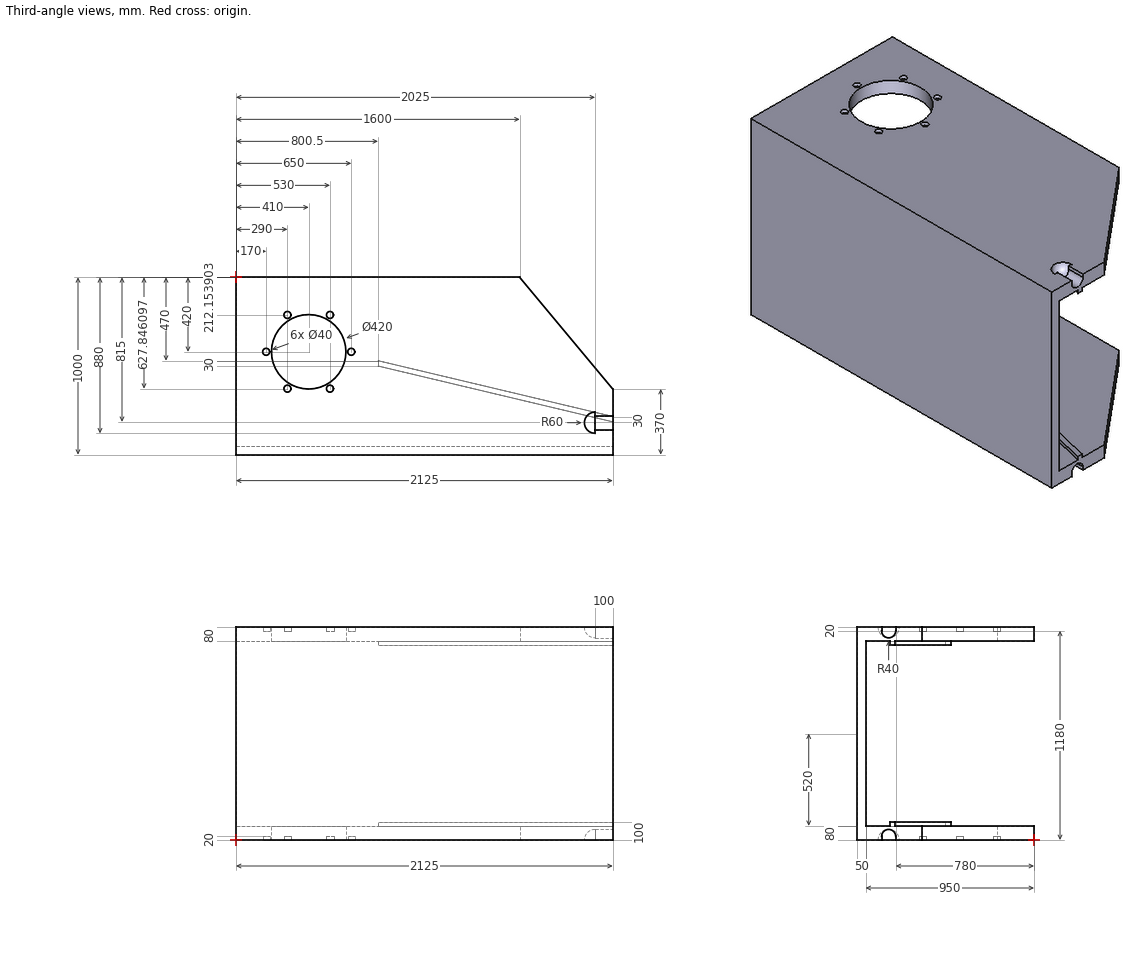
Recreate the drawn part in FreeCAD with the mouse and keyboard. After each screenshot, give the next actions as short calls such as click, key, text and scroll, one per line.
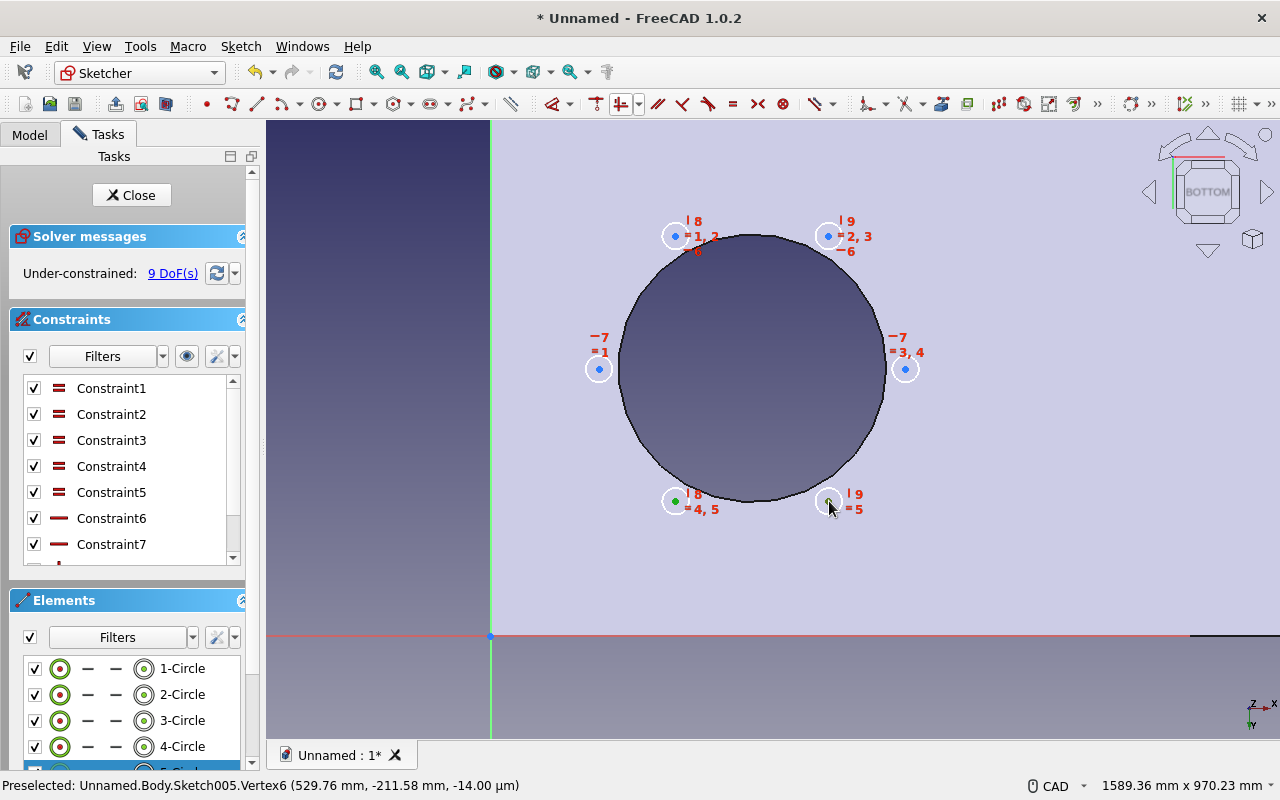
click(638, 104)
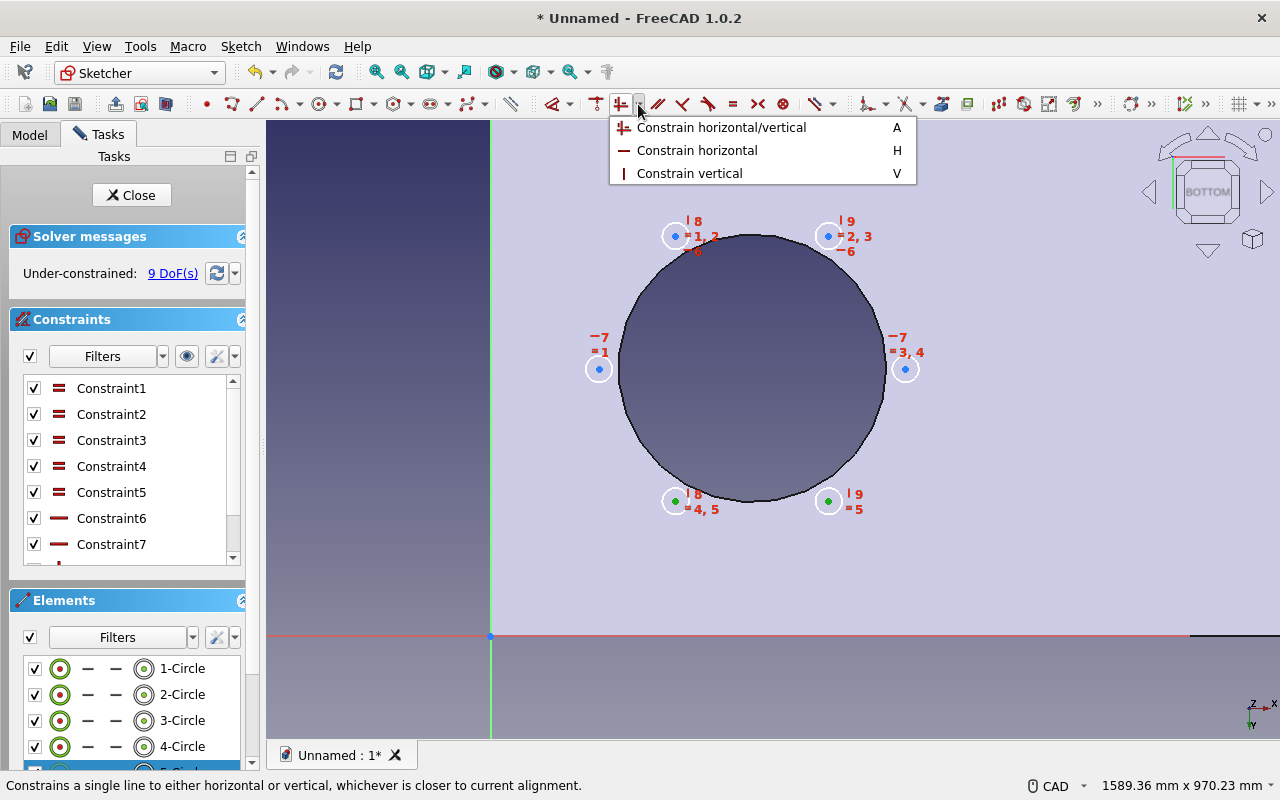
click(763, 150)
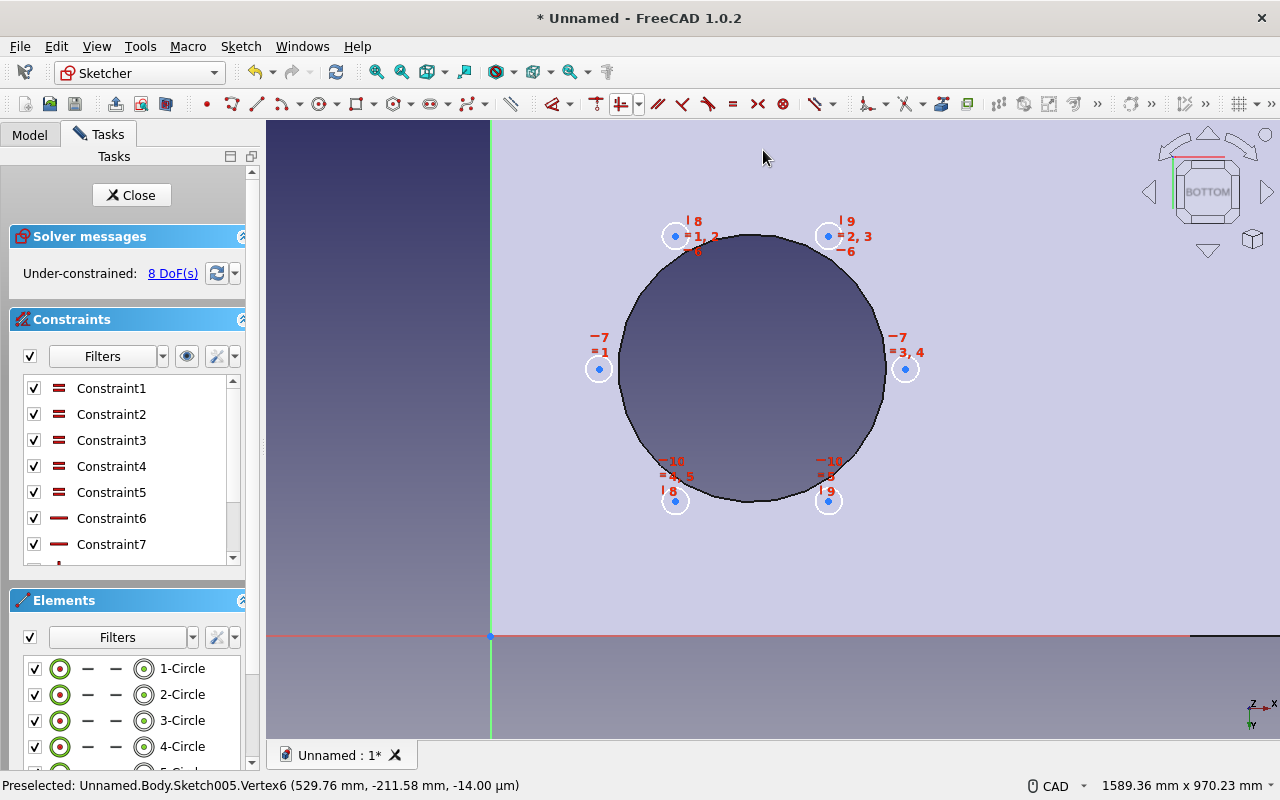
key(d)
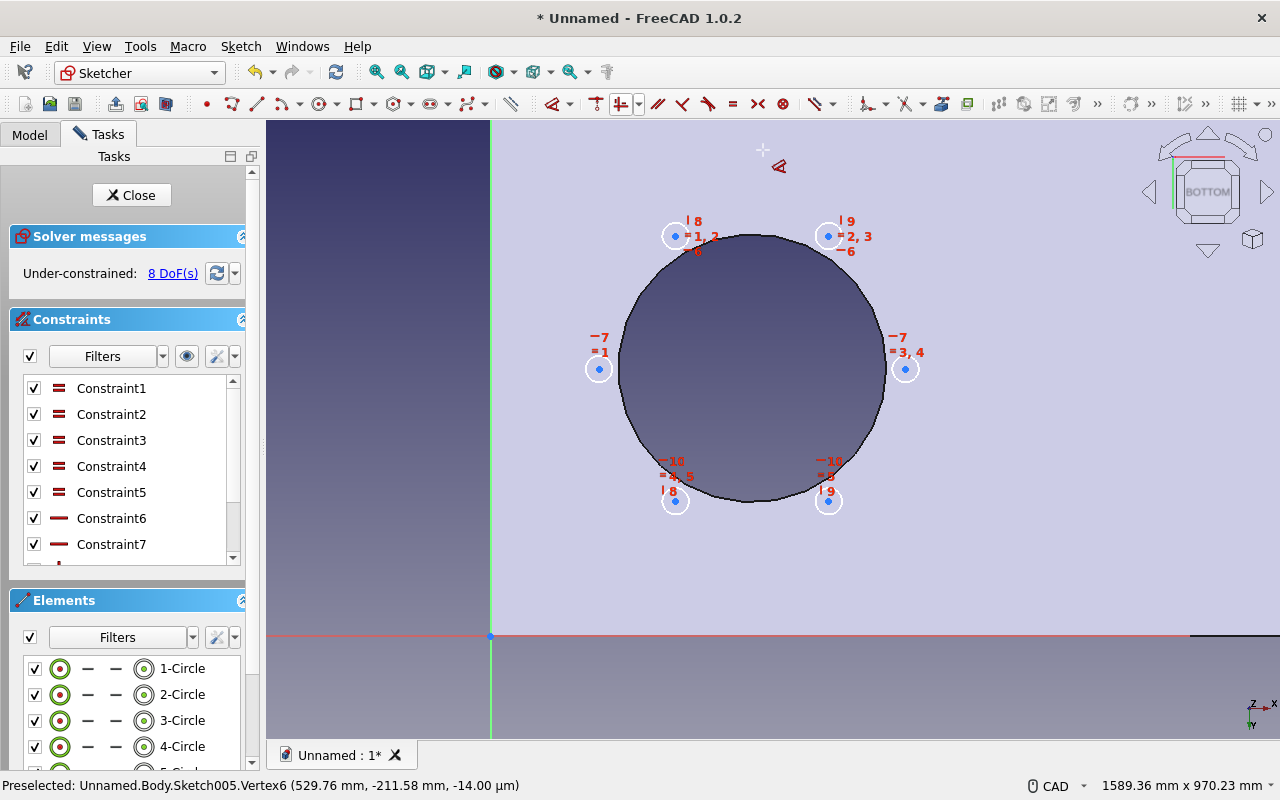
scroll(608, 360, up, 3)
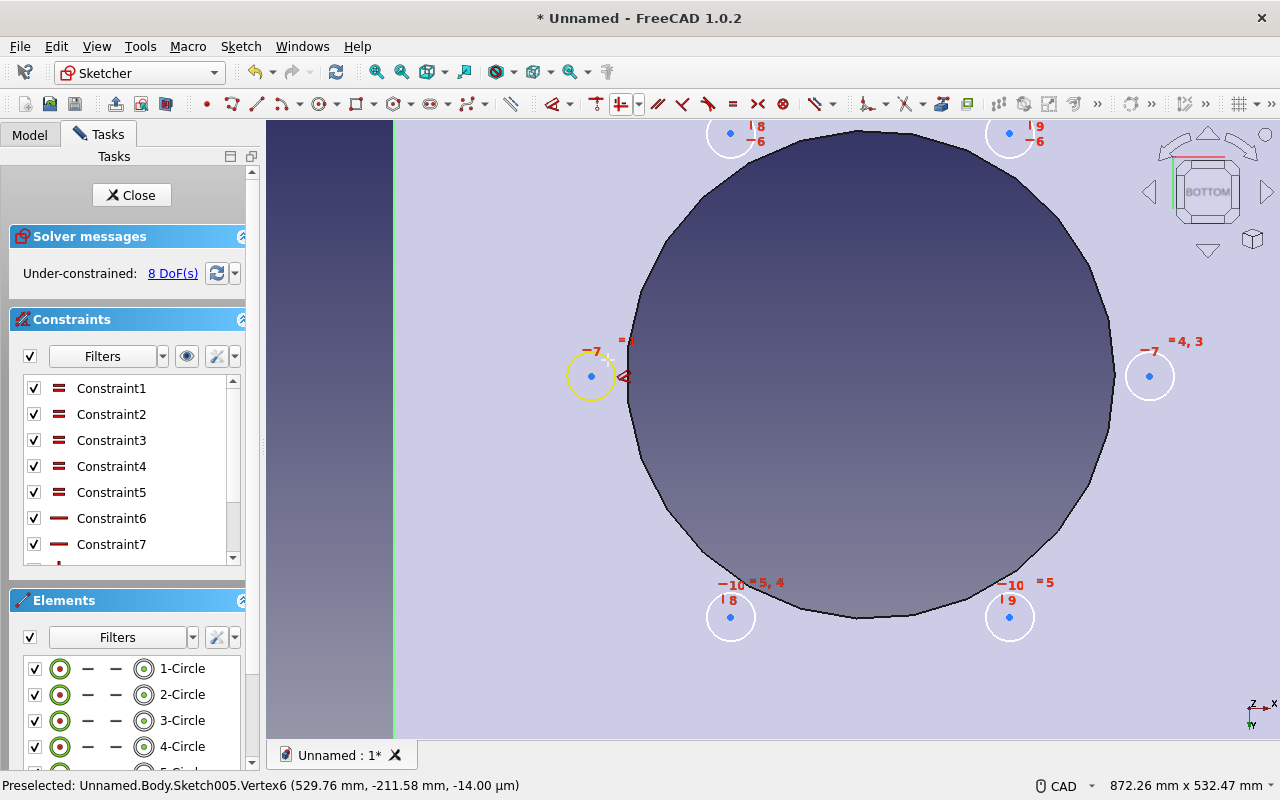
click(608, 359)
click(630, 336)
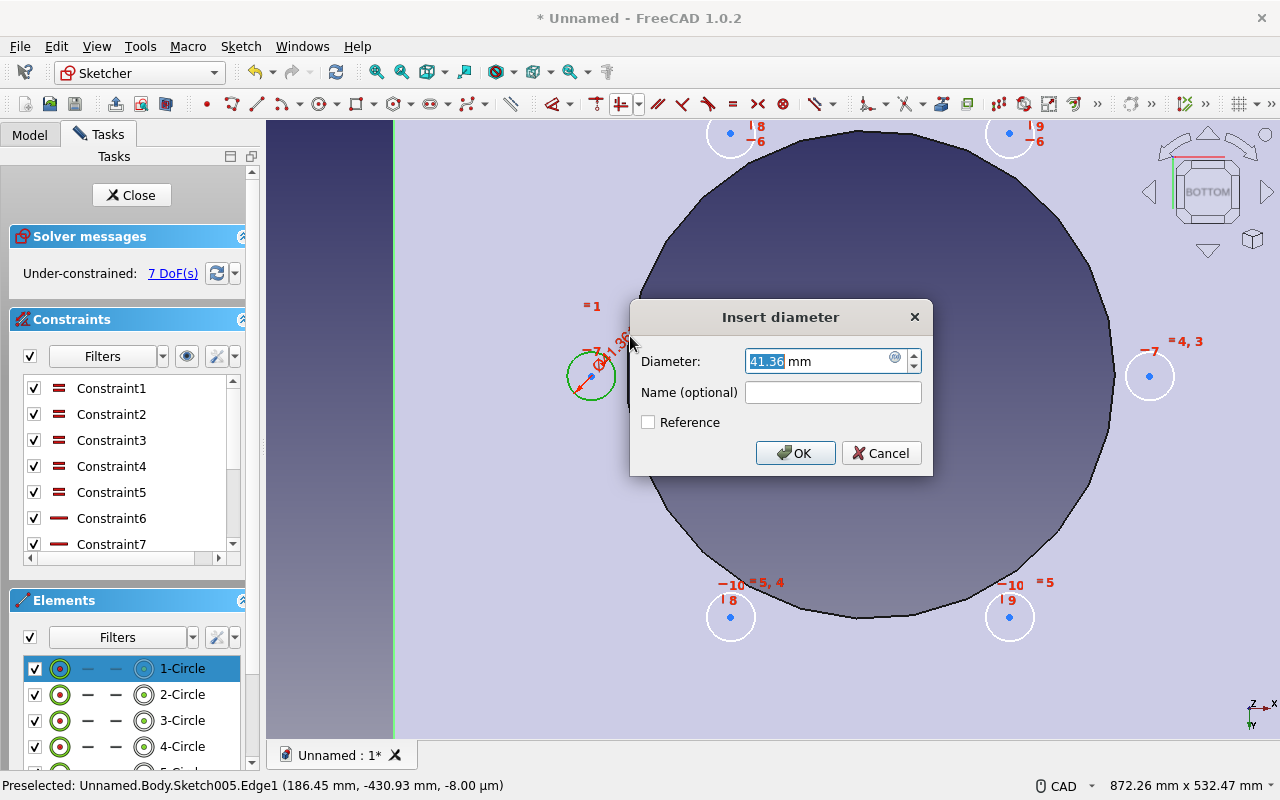
text(40)
key(Return)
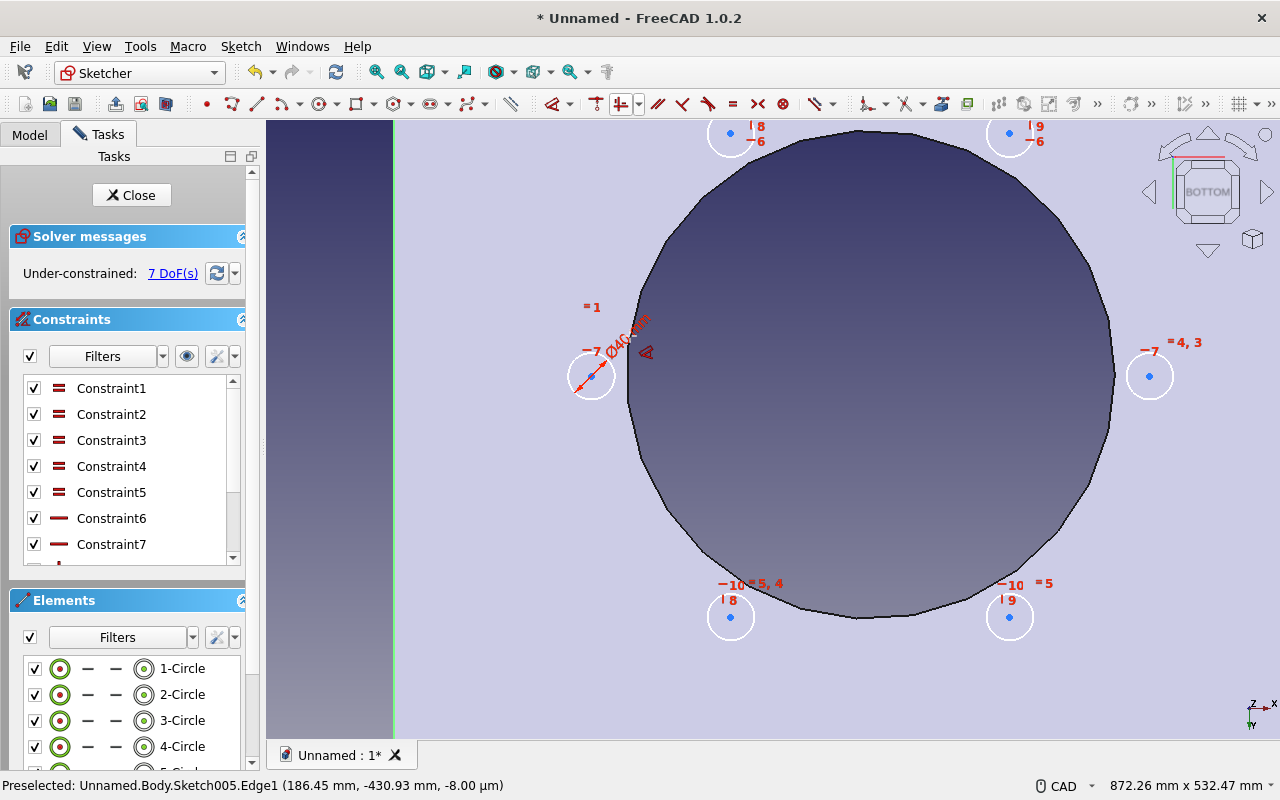
click(591, 376)
click(493, 342)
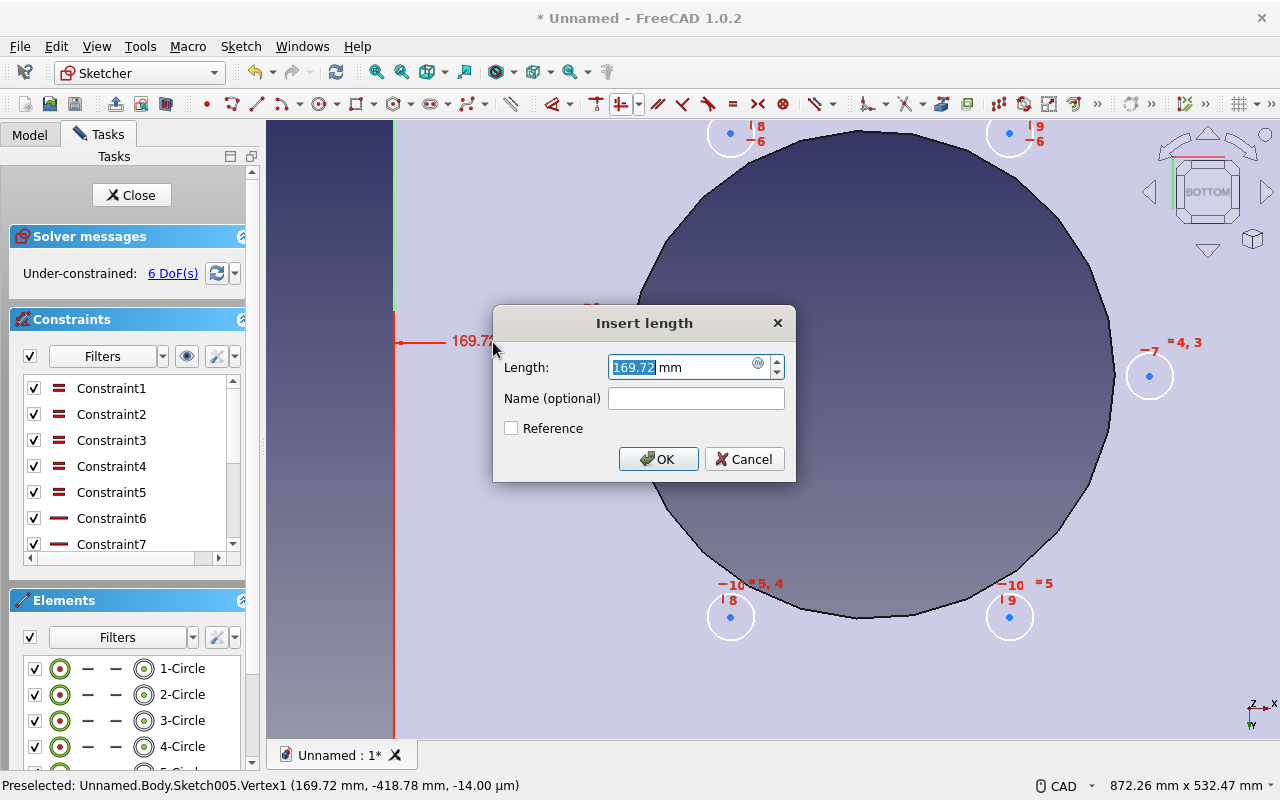
text(170)
key(Return)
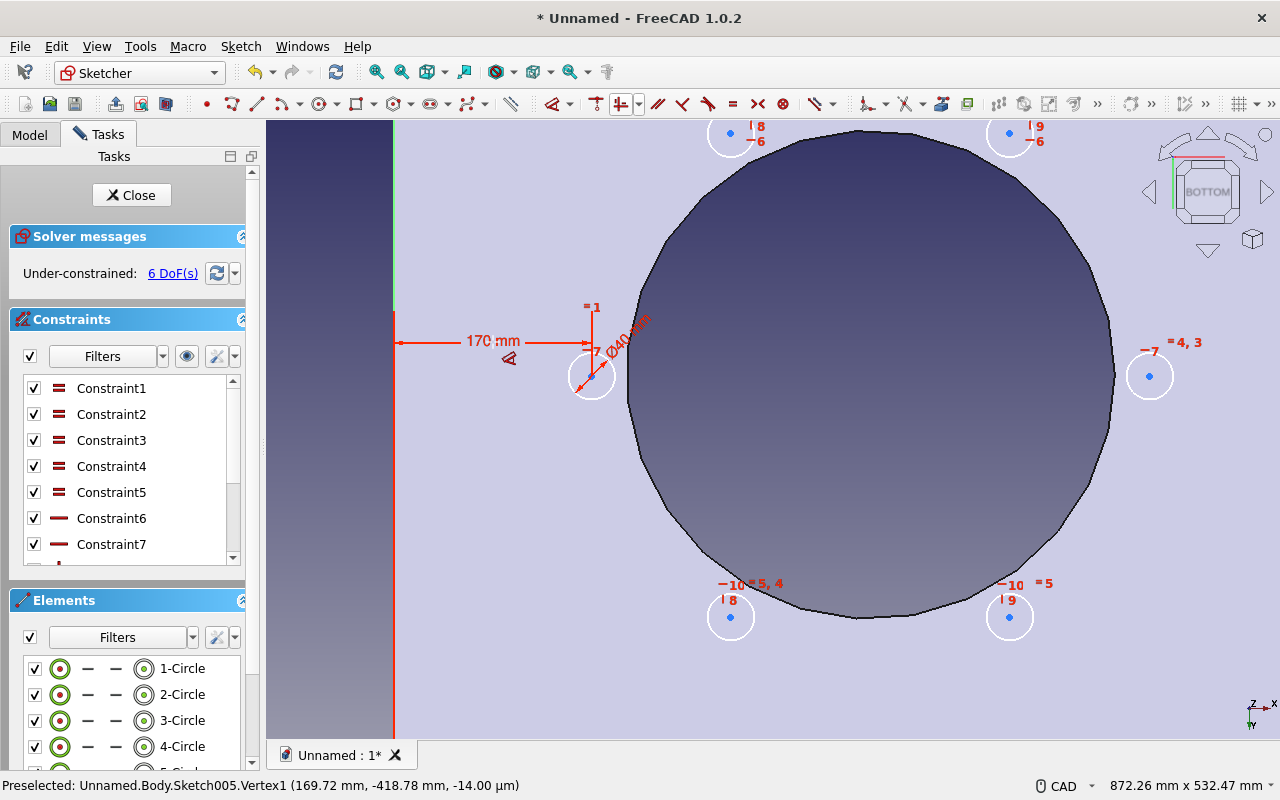
click(592, 376)
click(360, 544)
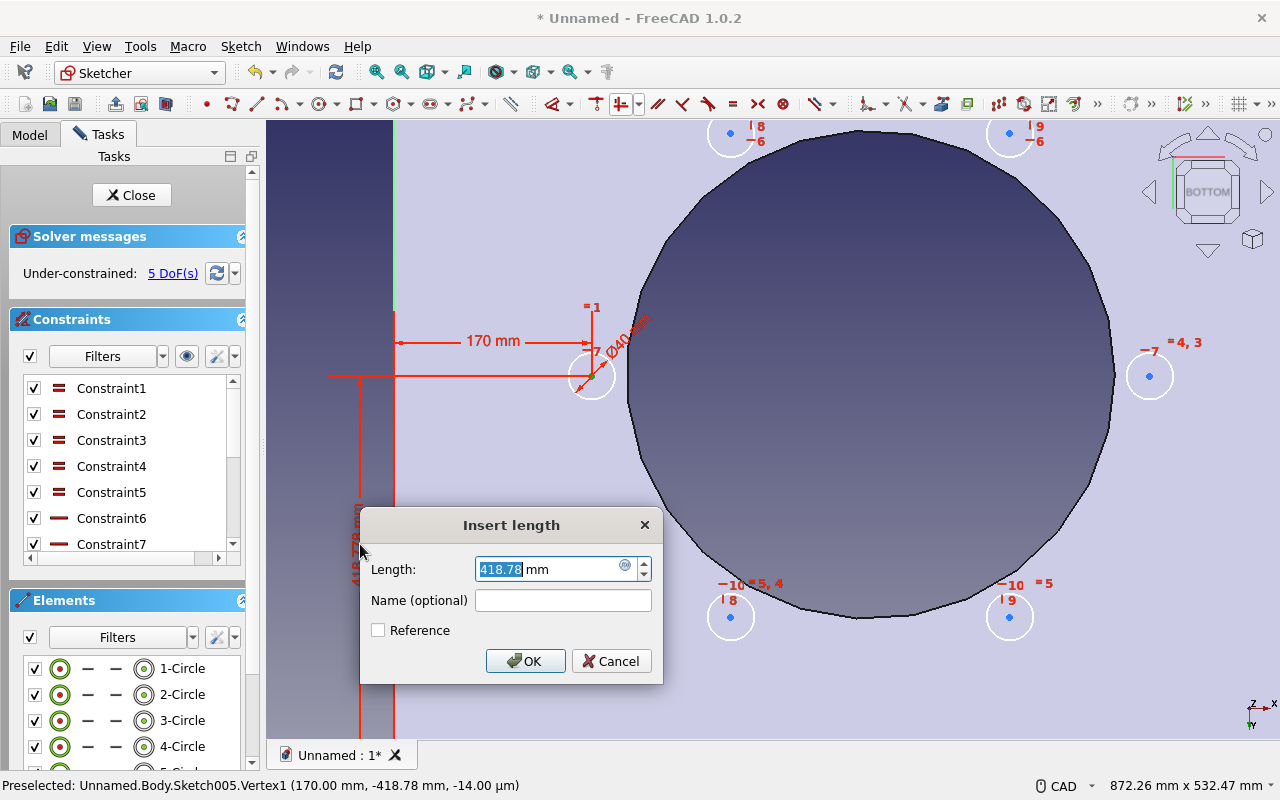
text(420)
key(Return)